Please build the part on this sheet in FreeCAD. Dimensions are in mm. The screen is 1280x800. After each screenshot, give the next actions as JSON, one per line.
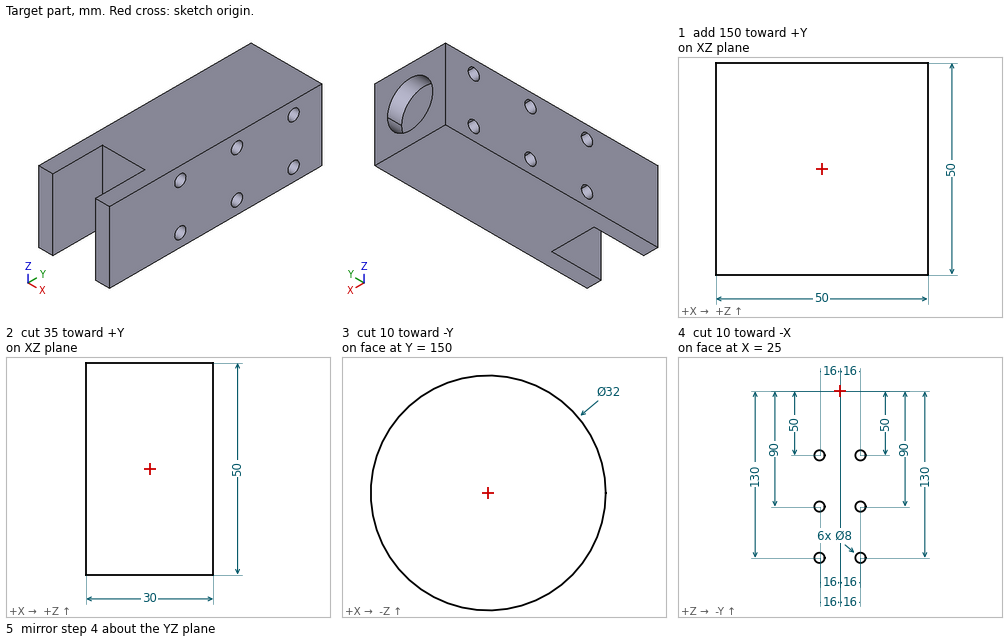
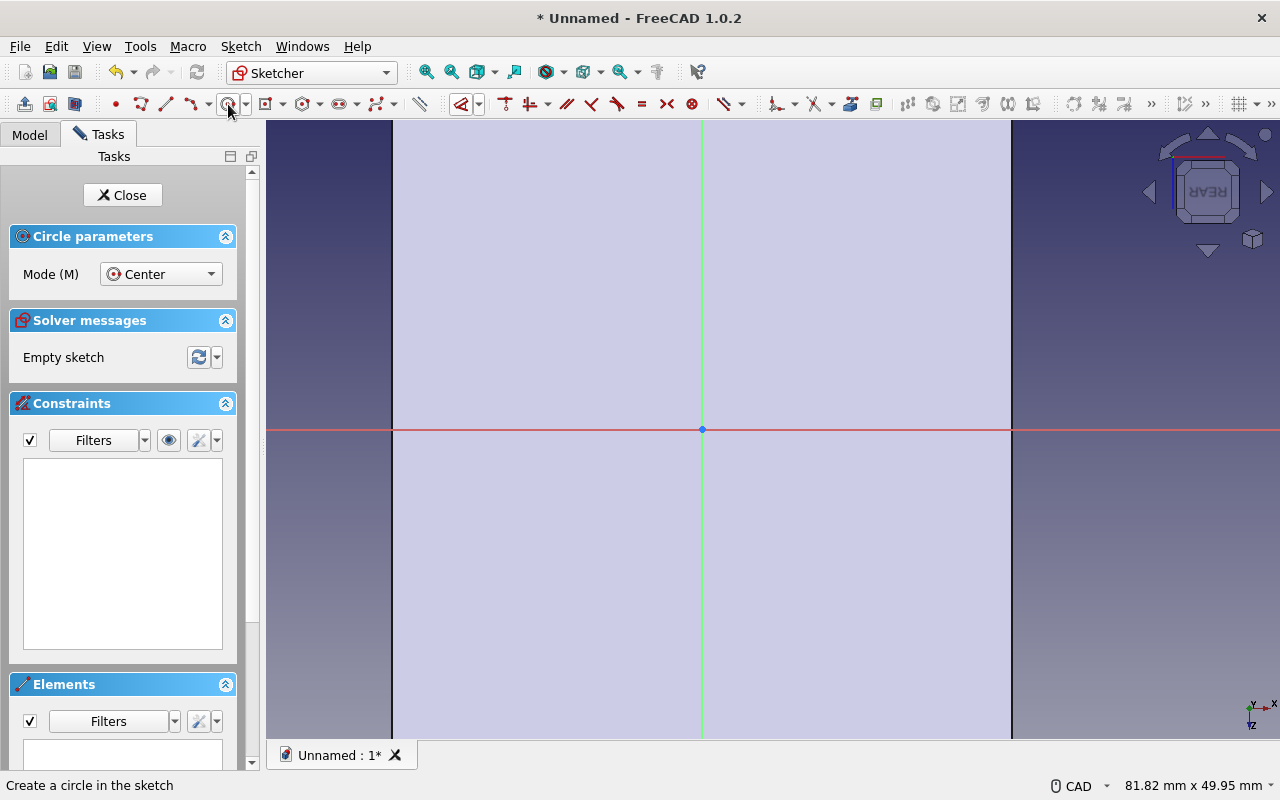
{"action": "left_click", "coordinate": [702, 429]}
{"action": "mouse_move", "coordinate": [842, 289]}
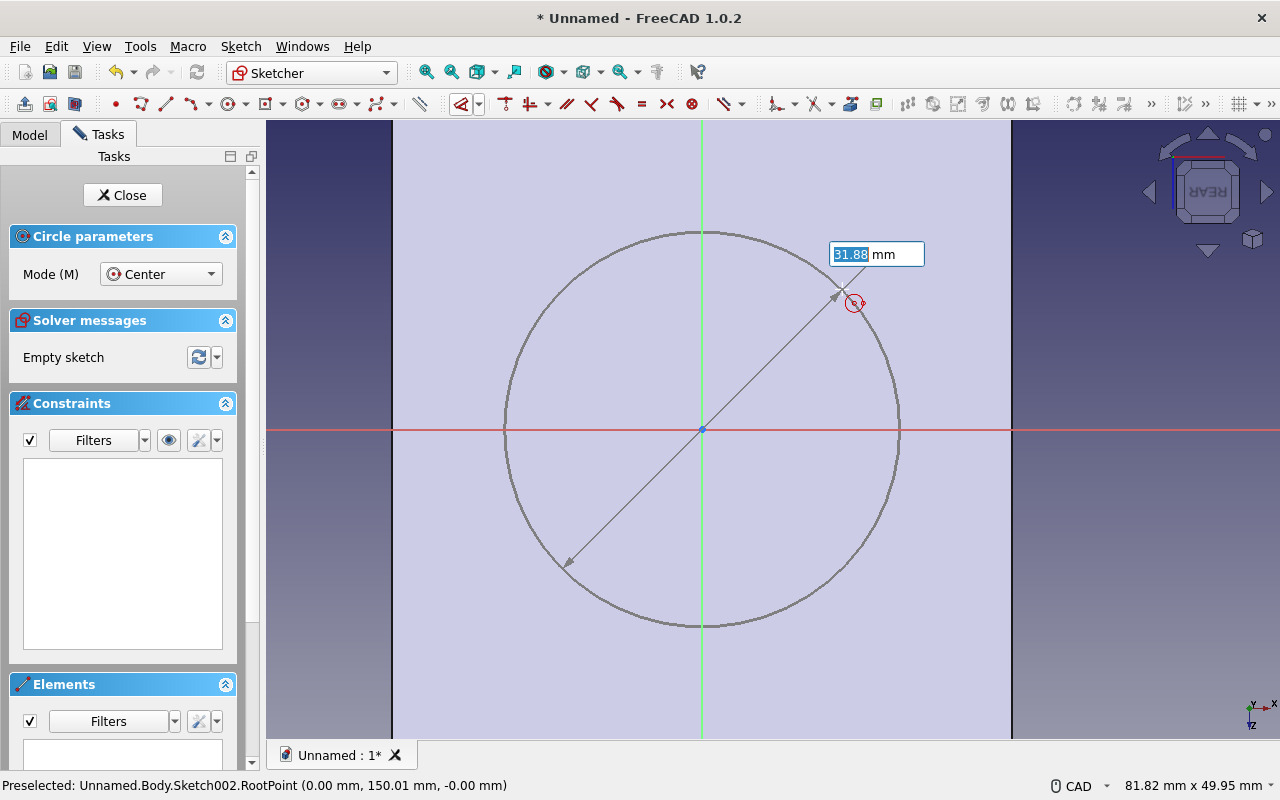
{"action": "type", "text": "32"}
{"action": "key", "text": "Return"}
{"action": "key", "text": "Escape"}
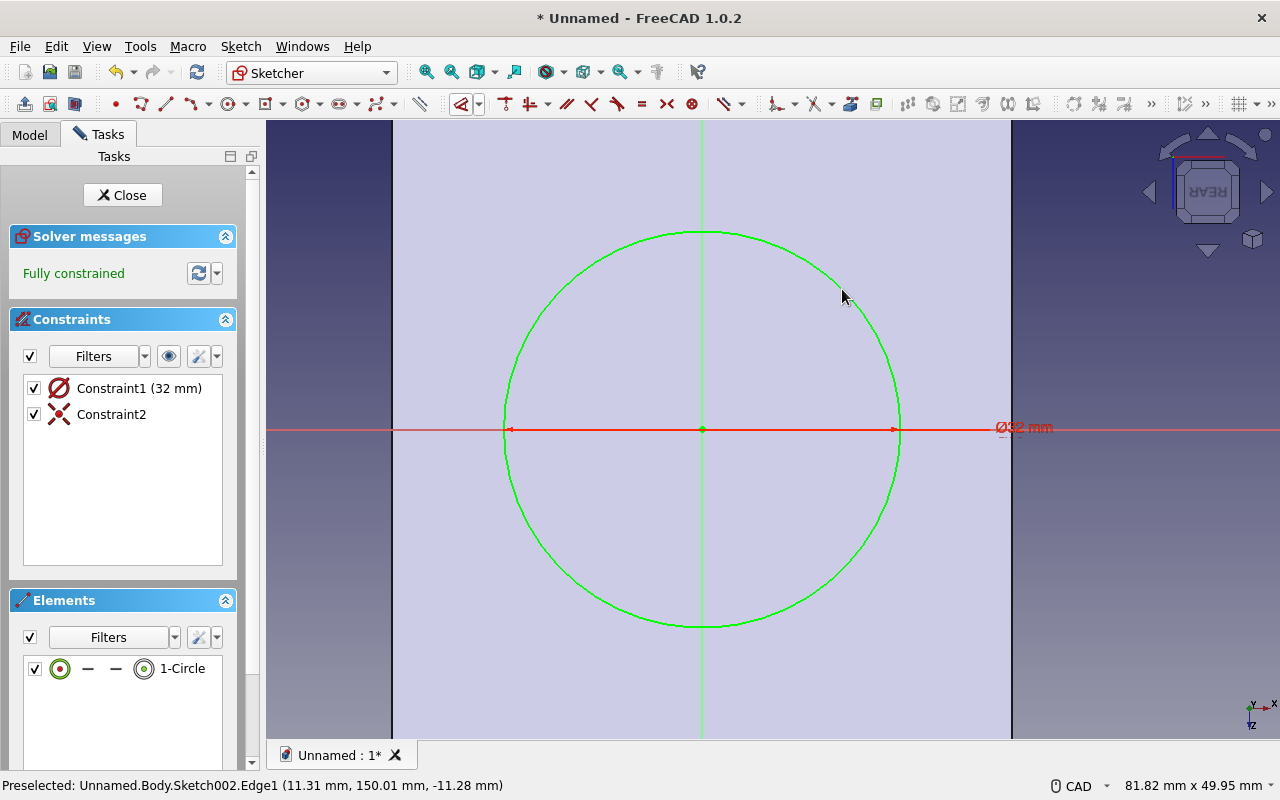
{"action": "left_click", "coordinate": [123, 195]}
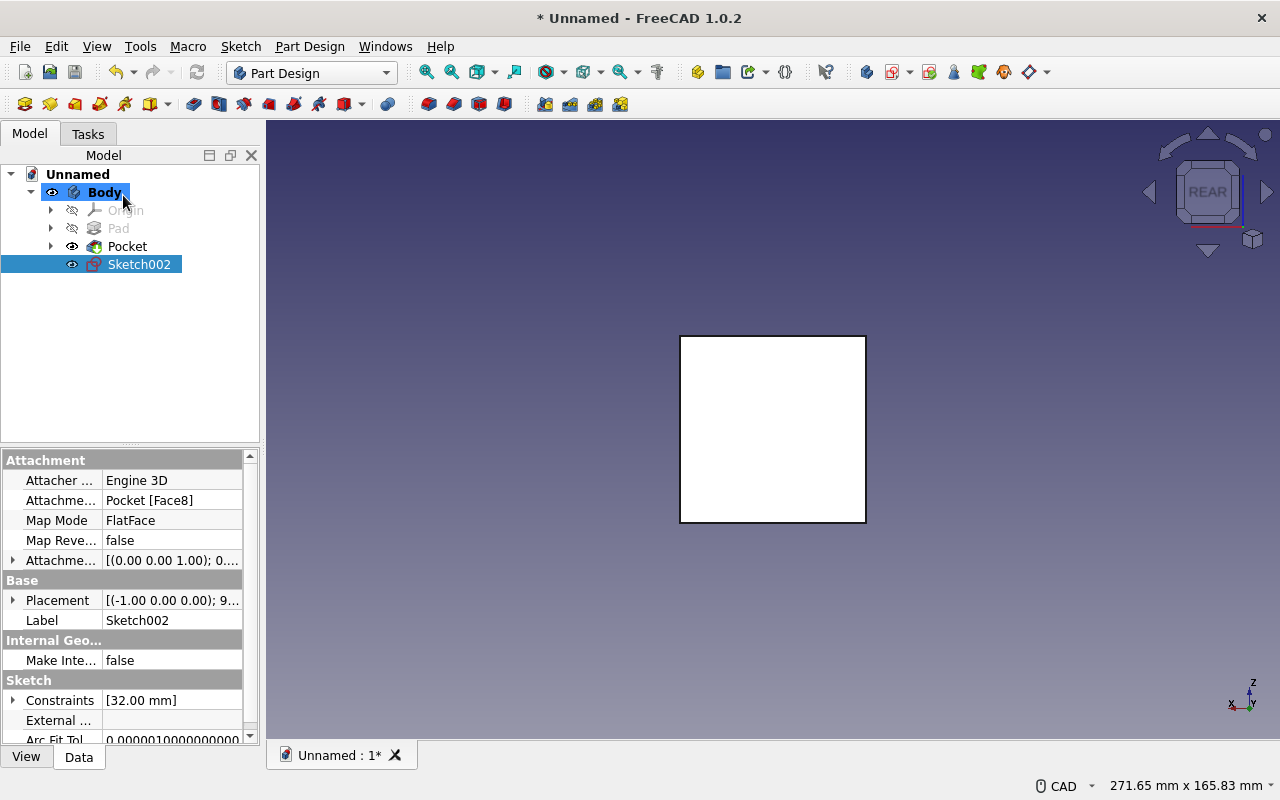
{"action": "left_click", "coordinate": [194, 104]}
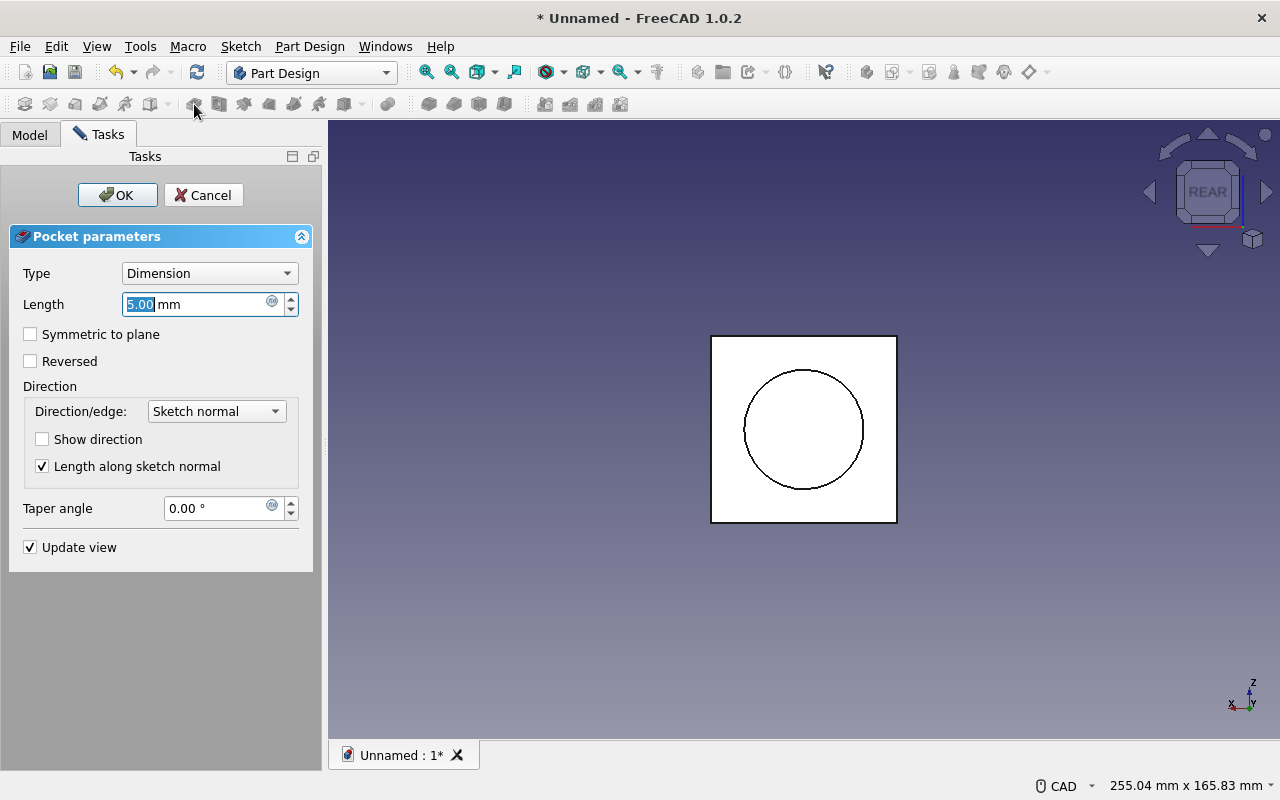
{"action": "type", "text": "10"}
{"action": "key", "text": "Tab"}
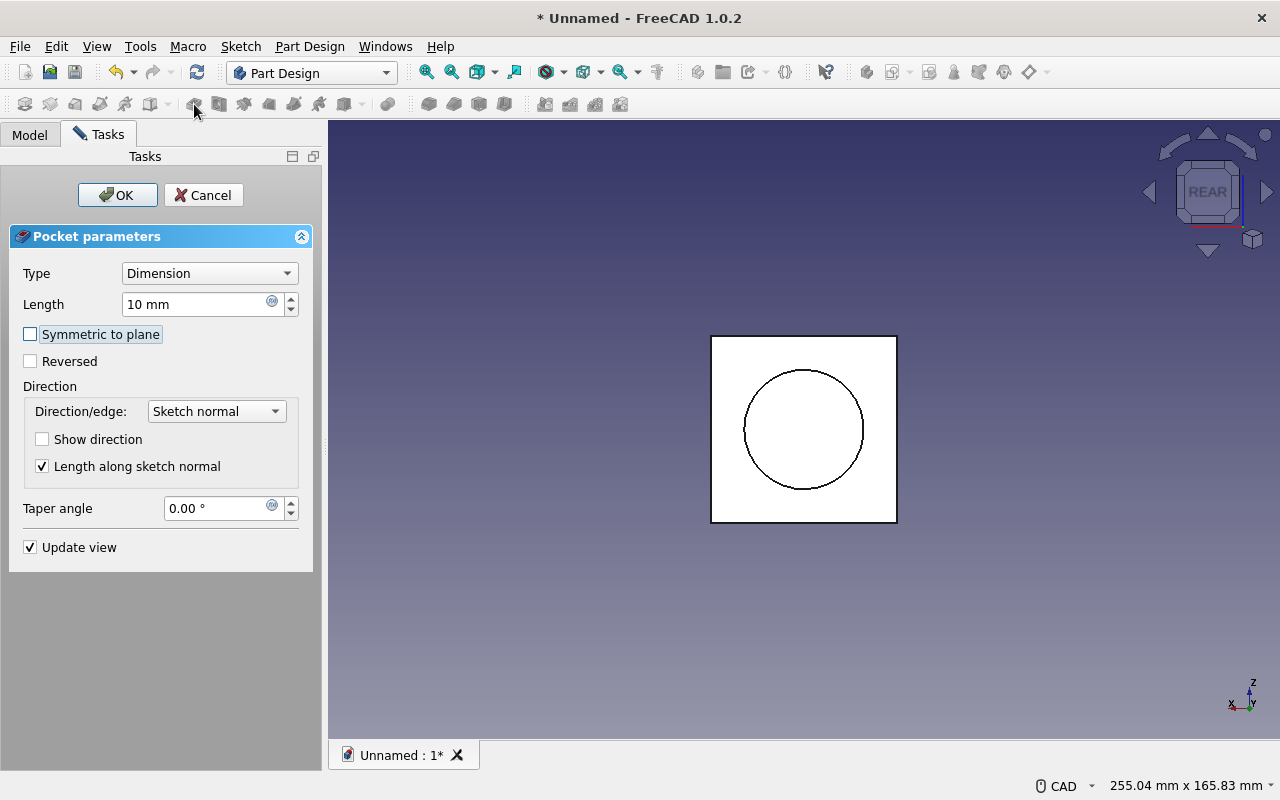
{"action": "left_click", "coordinate": [118, 195]}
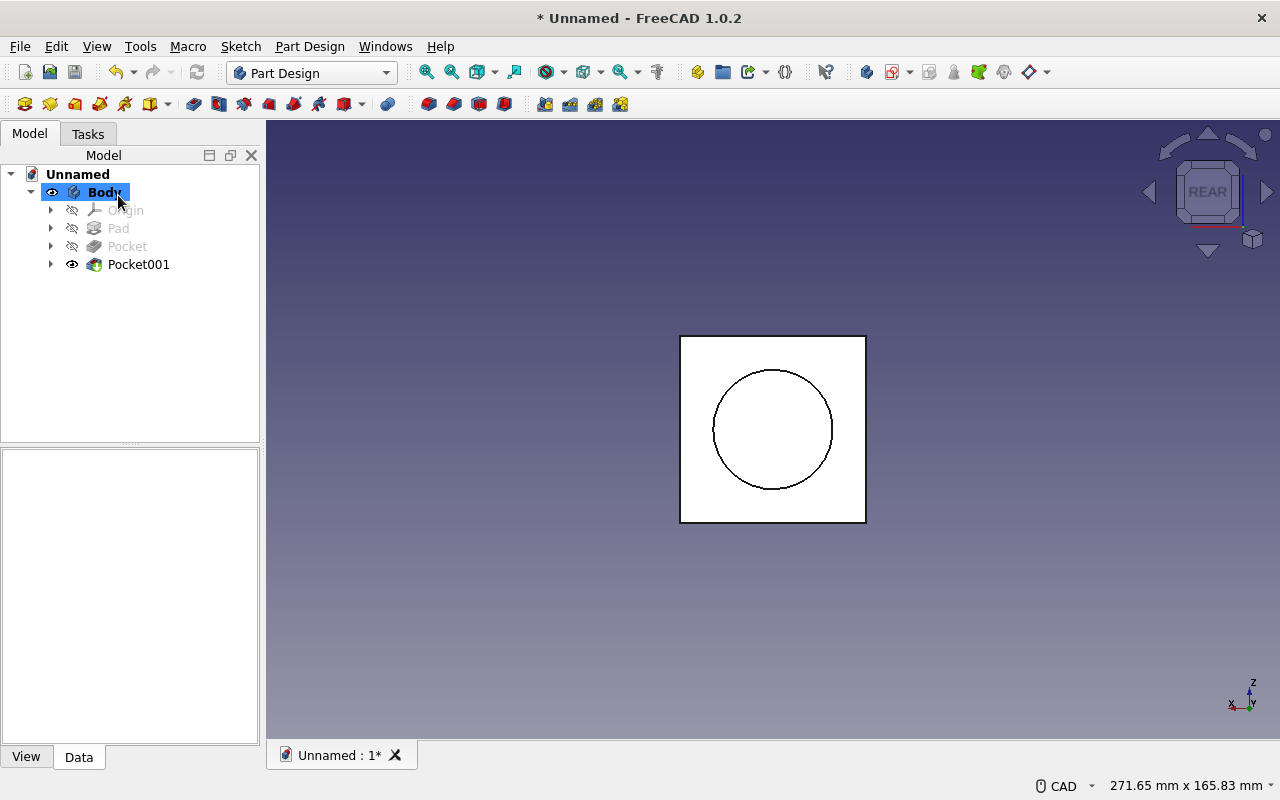
{"action": "left_click", "coordinate": [427, 72]}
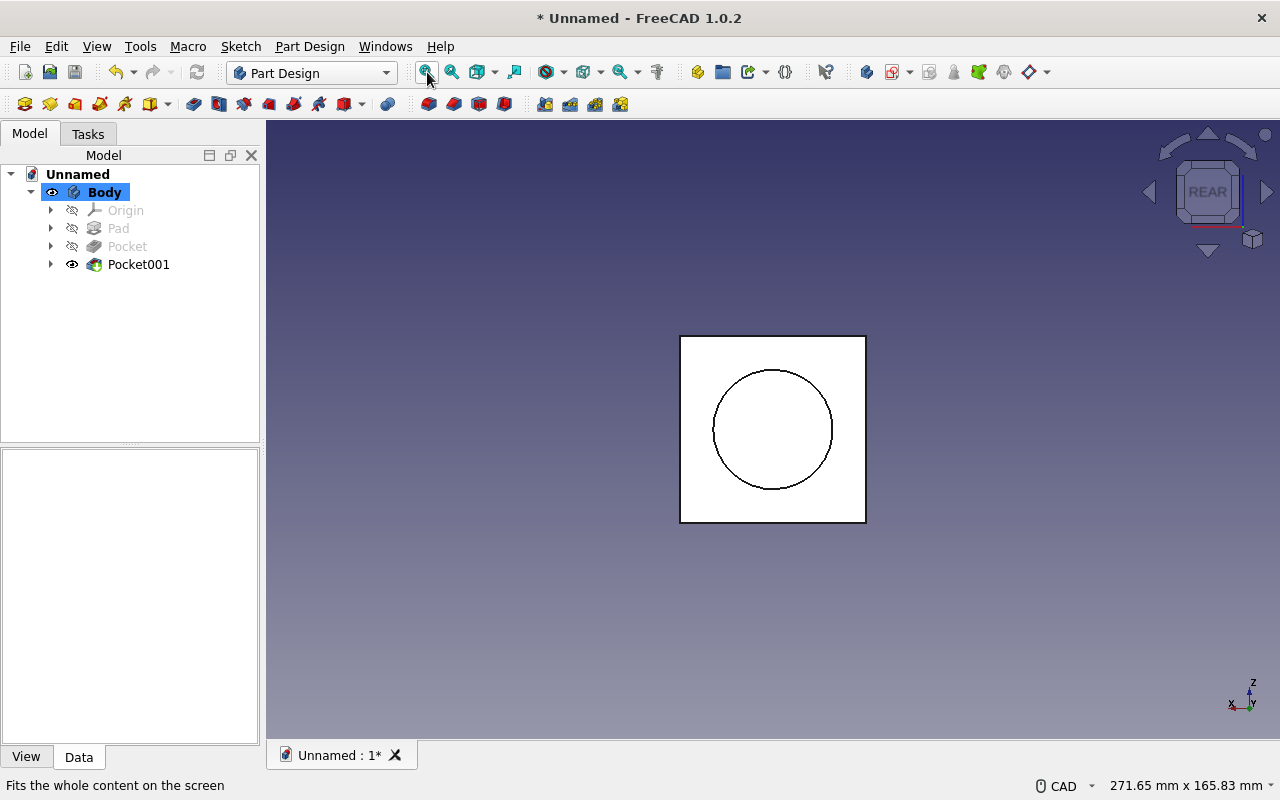
{"action": "key", "text": "0"}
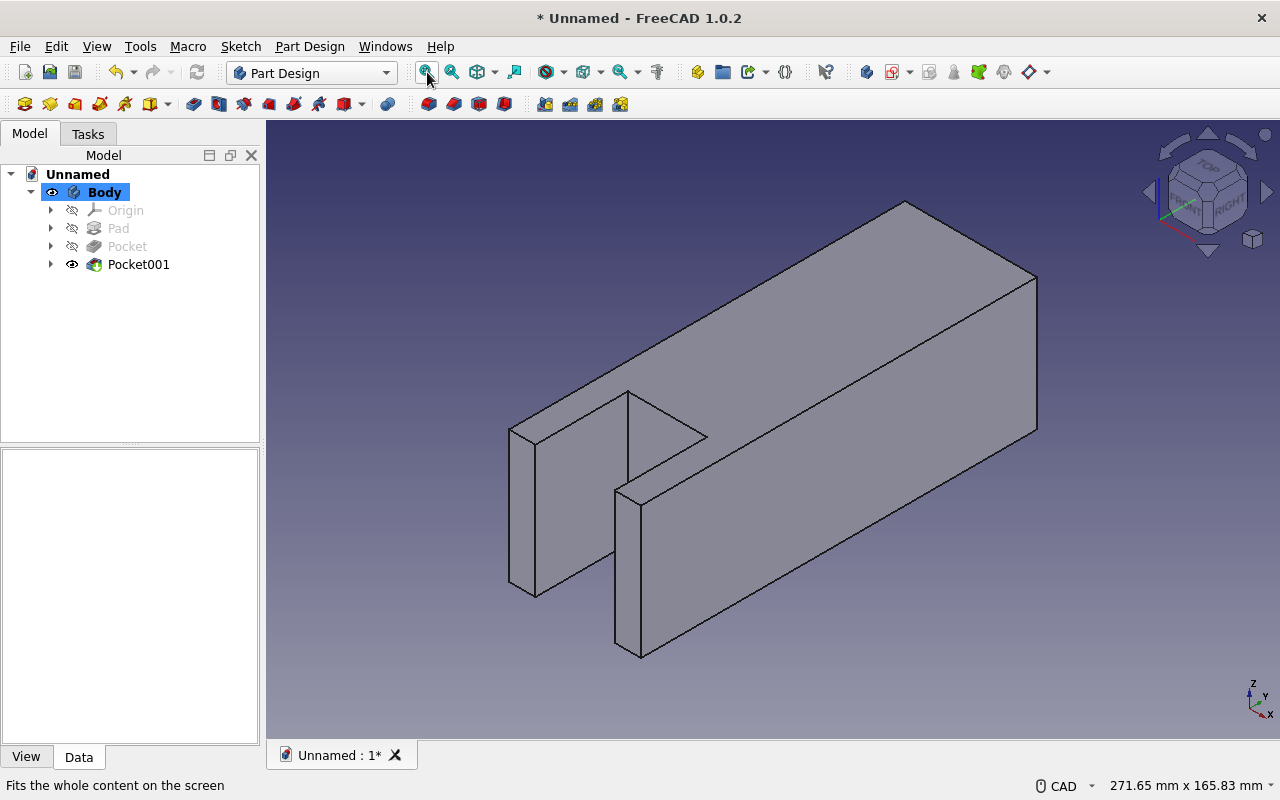
{"action": "left_click", "coordinate": [896, 434]}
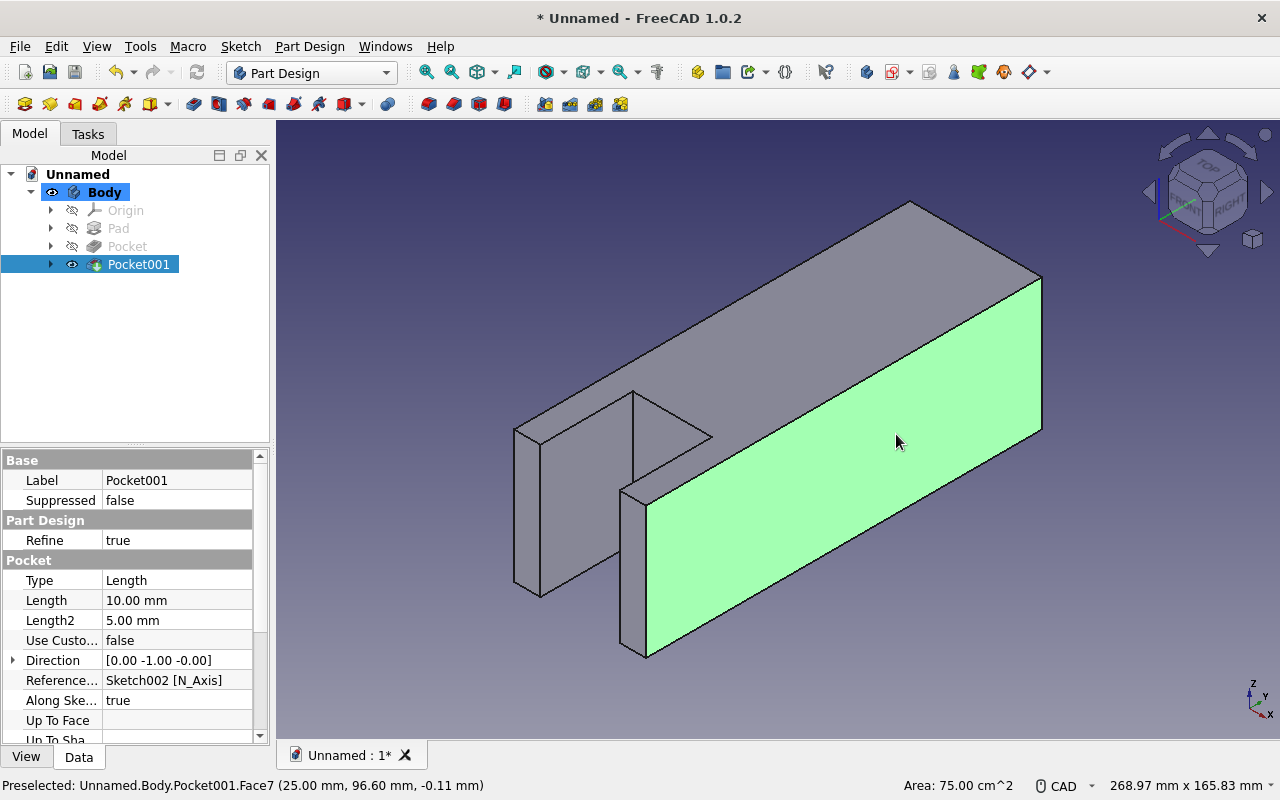
{"action": "left_click", "coordinate": [892, 72]}